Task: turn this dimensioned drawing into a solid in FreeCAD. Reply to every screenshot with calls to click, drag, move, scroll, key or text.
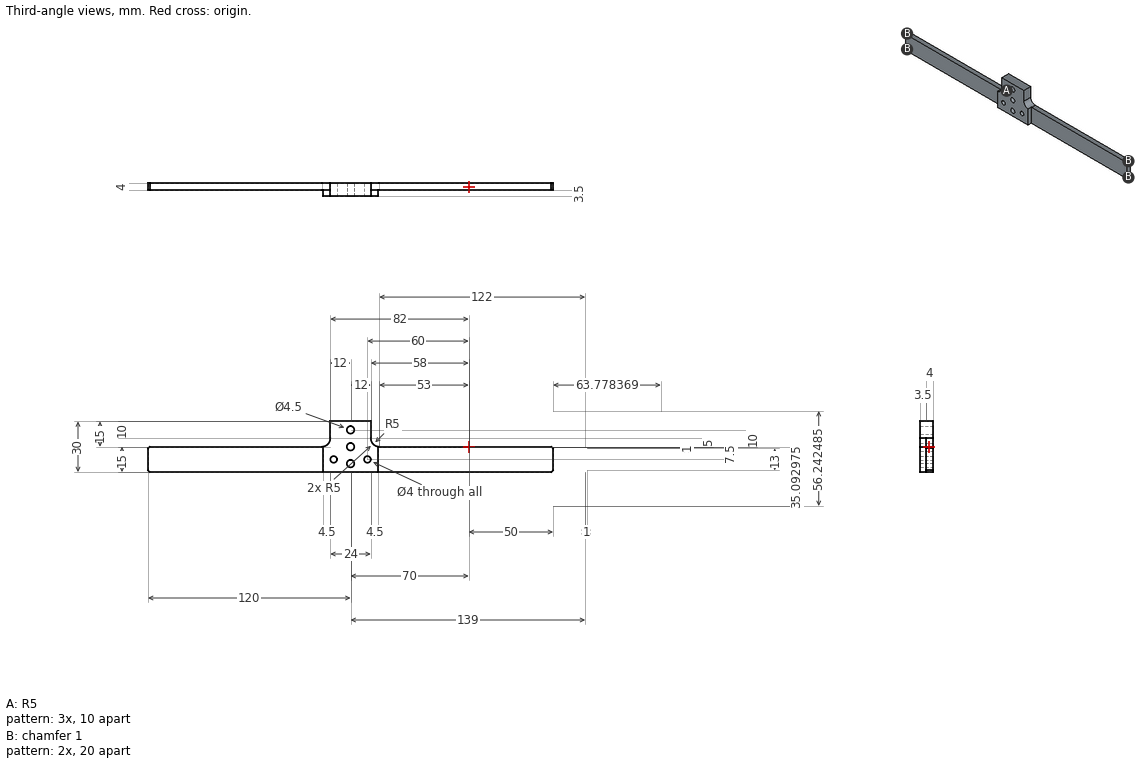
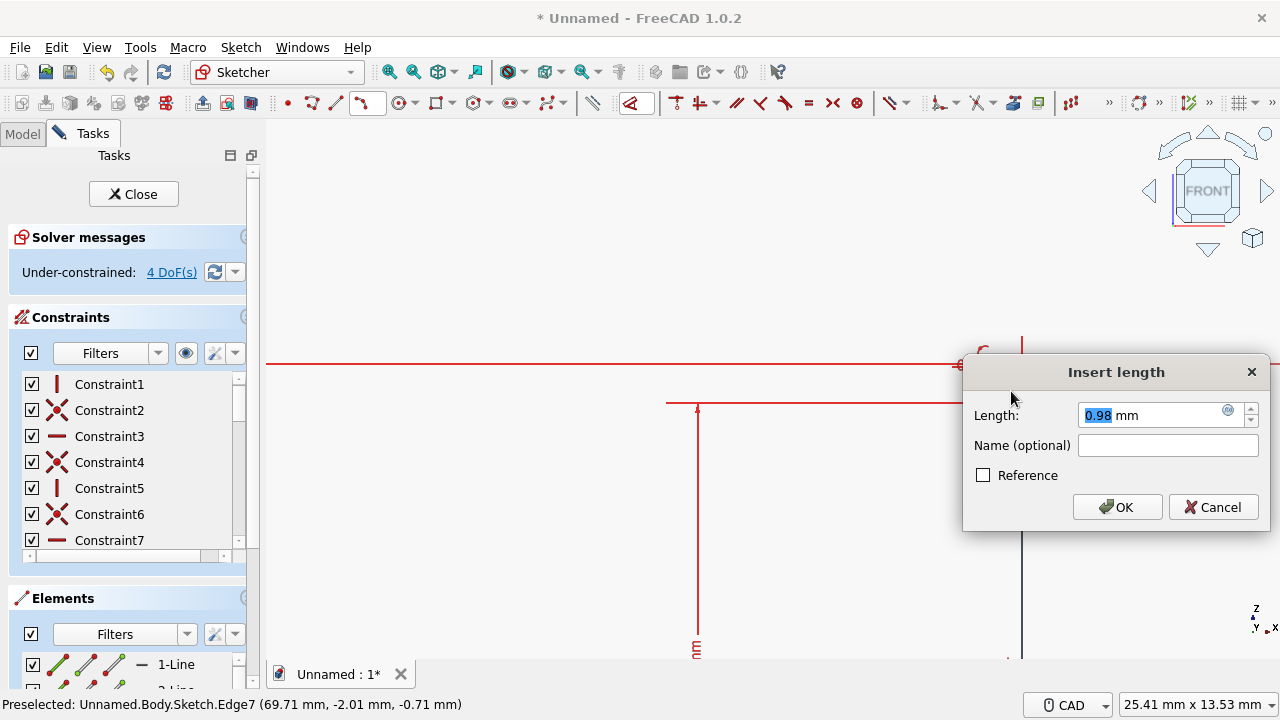
text(1)
key(Return)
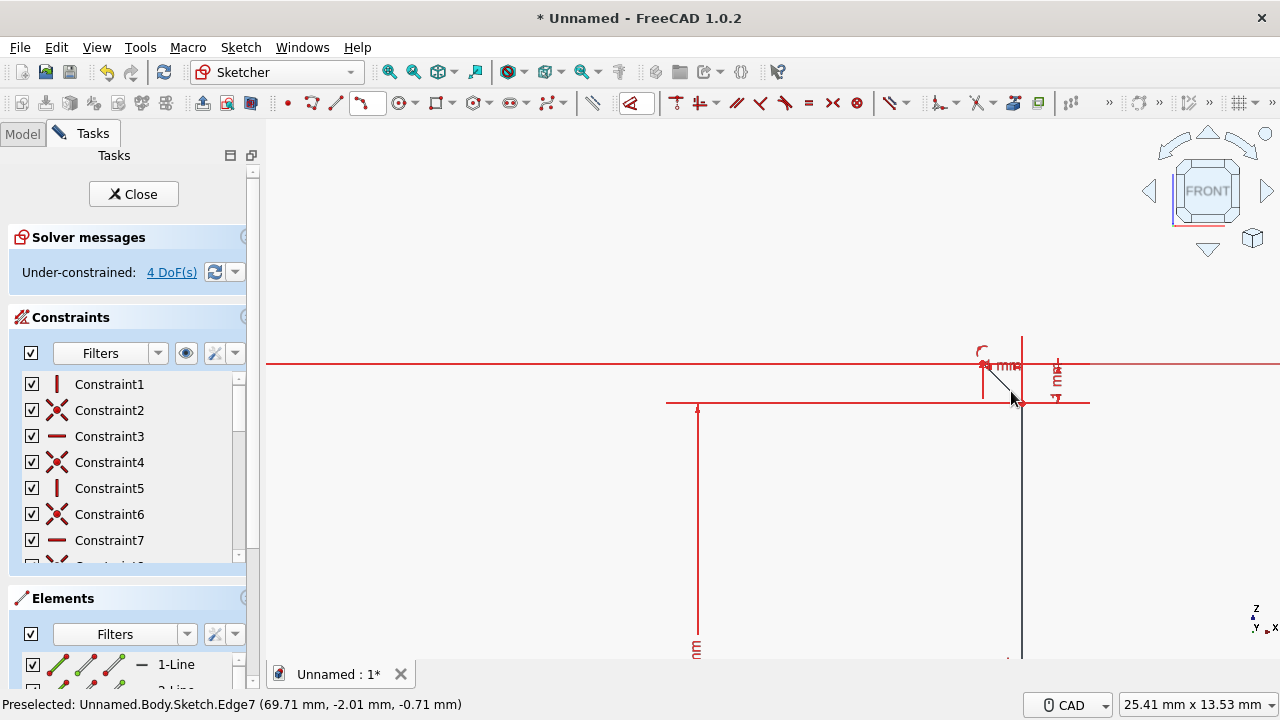
scroll(1013, 392, down, 11)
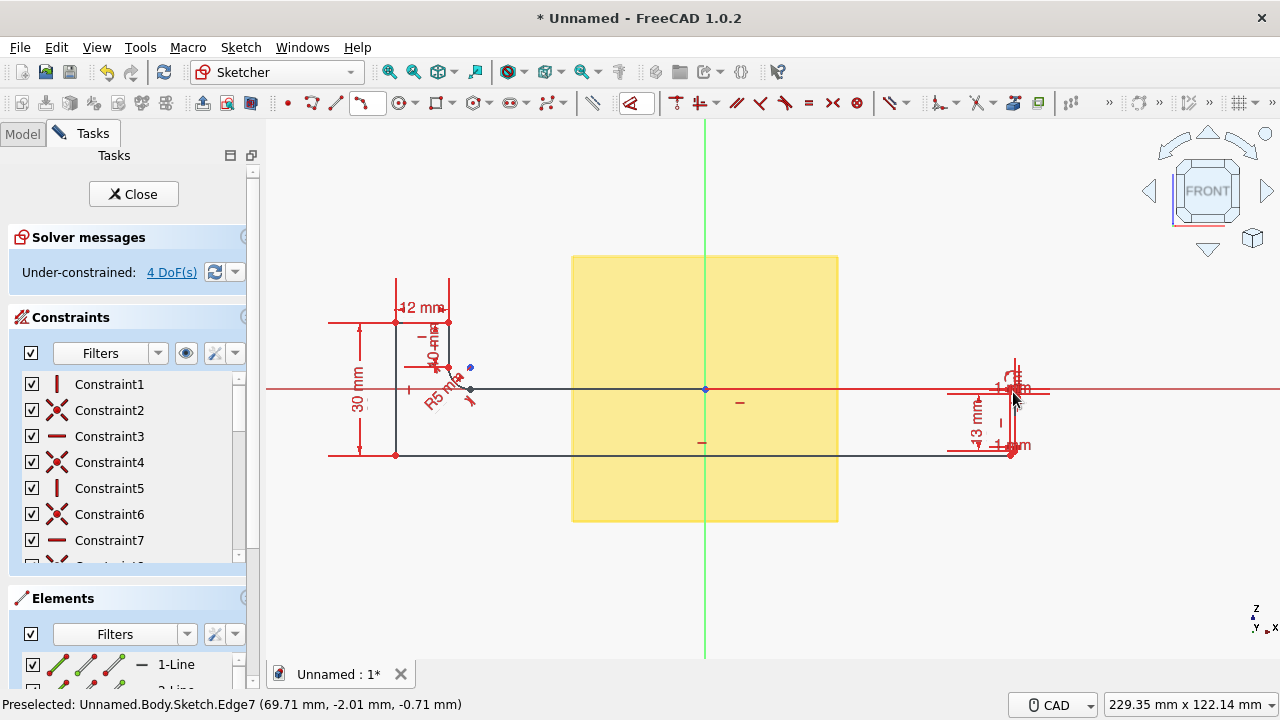
click(580, 456)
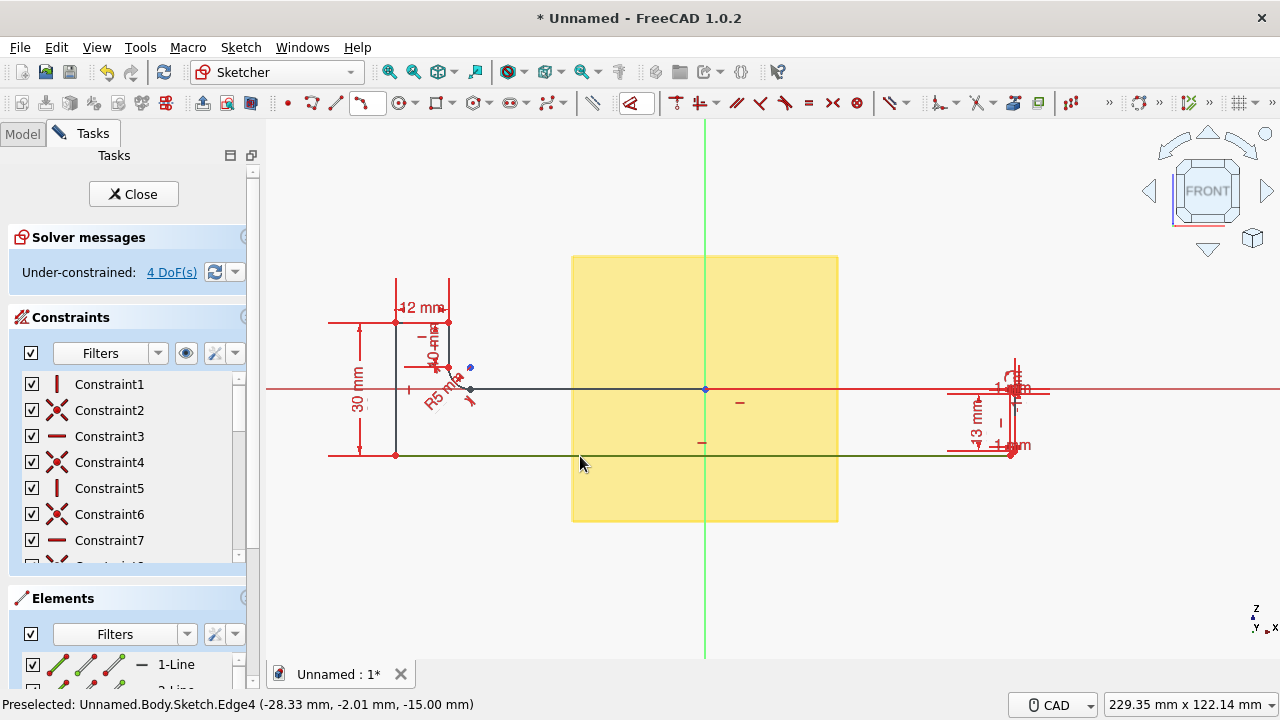
click(648, 104)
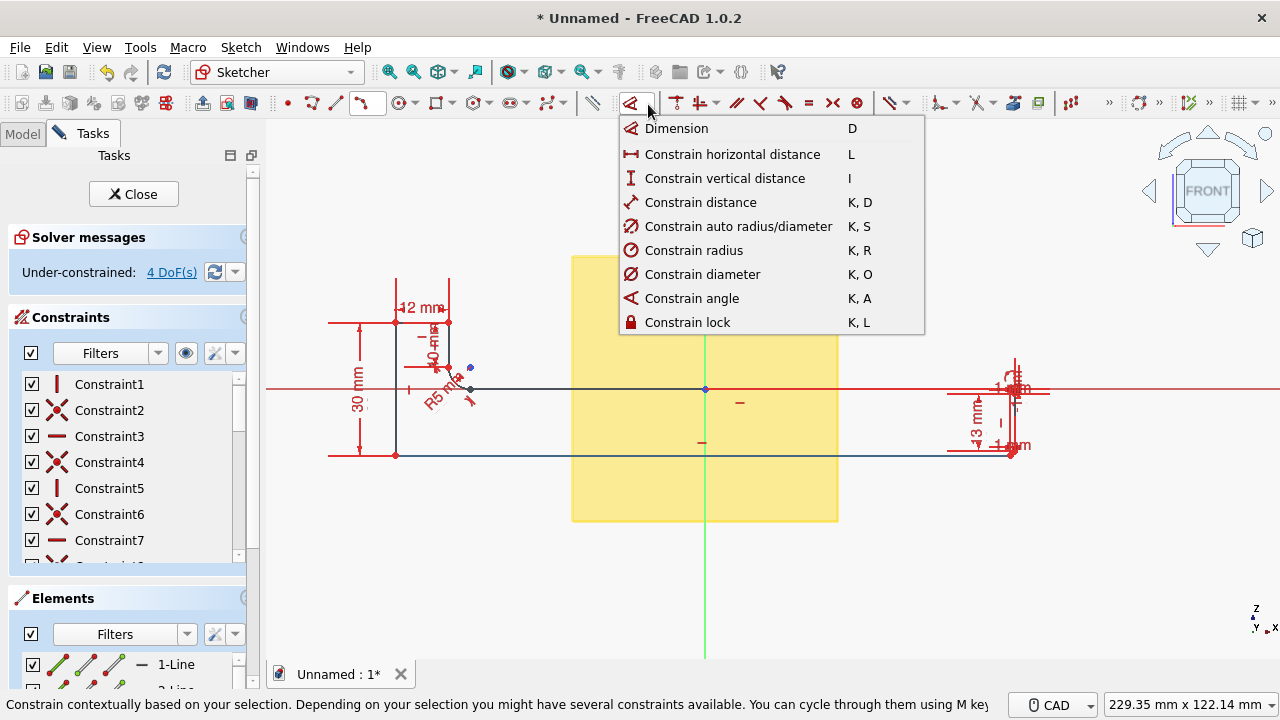
click(772, 154)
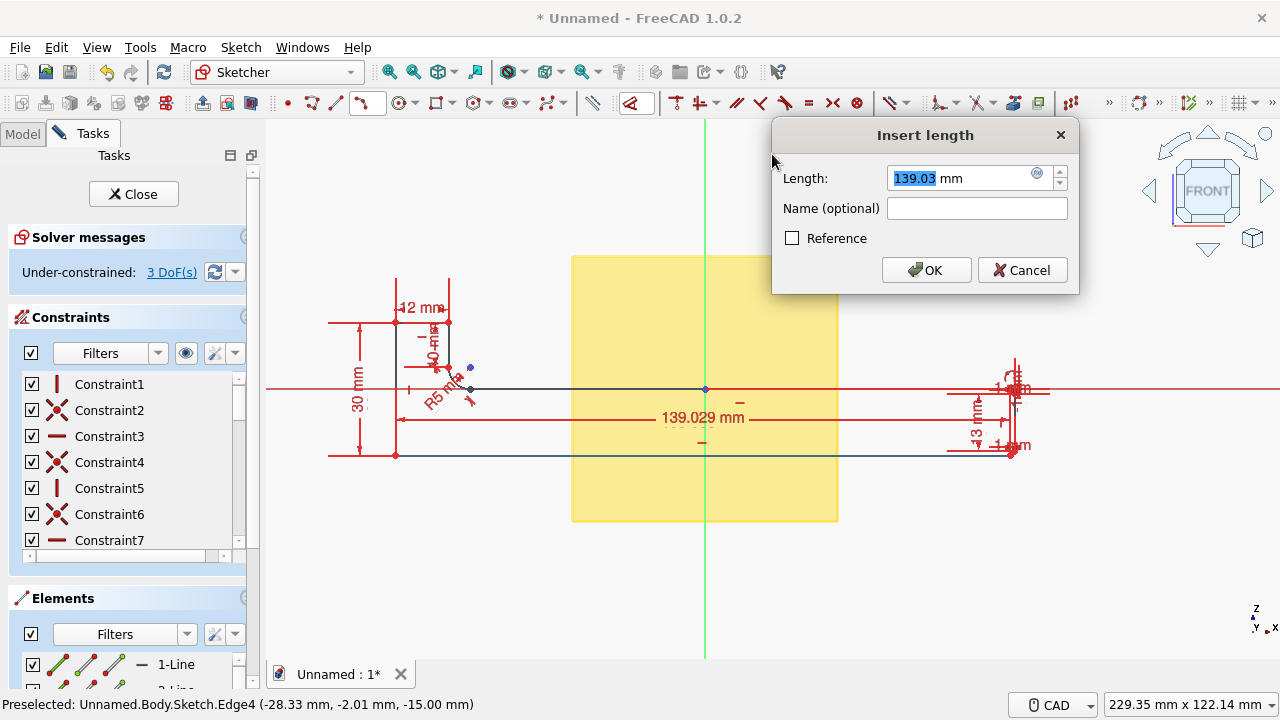
text(139)
key(Return)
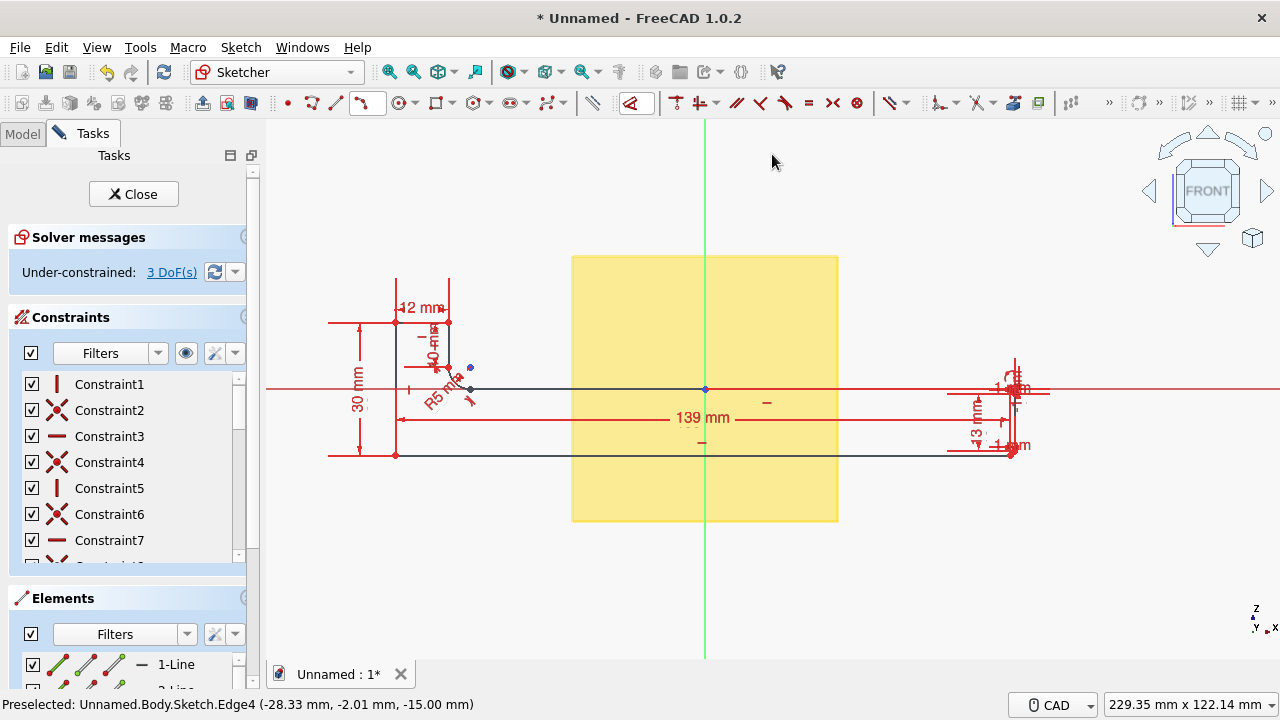
click(848, 389)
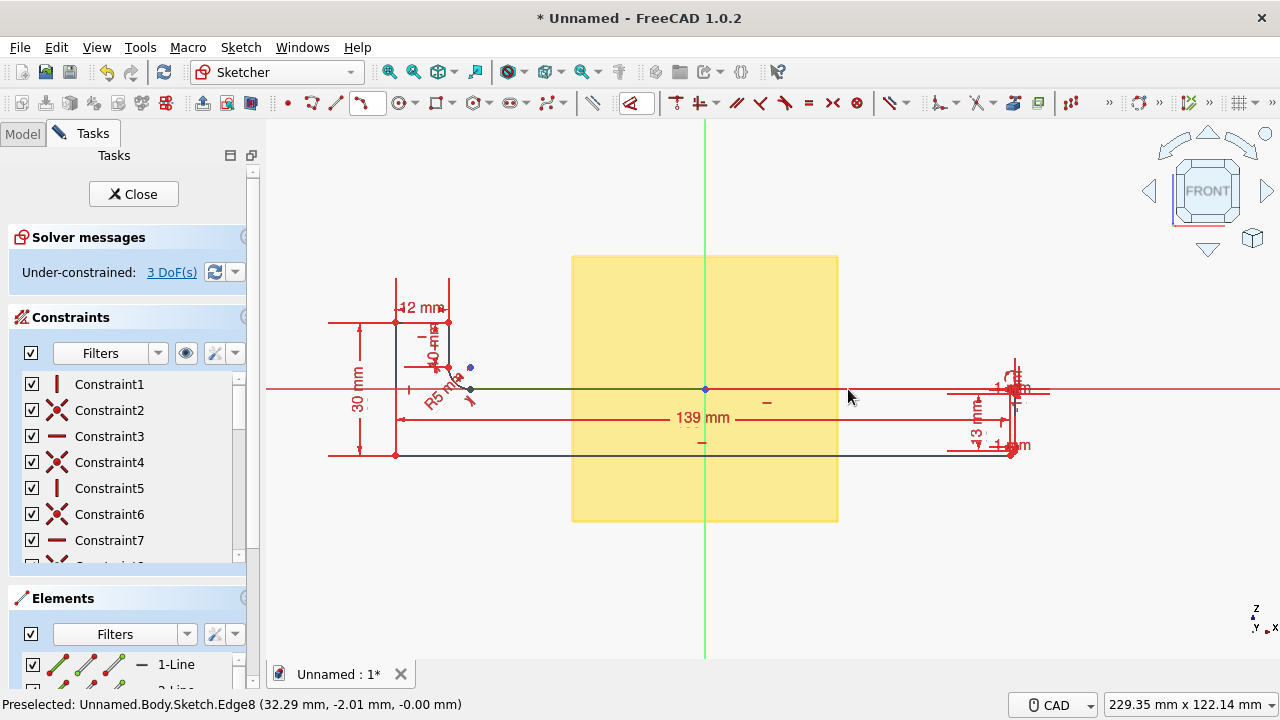
click(648, 104)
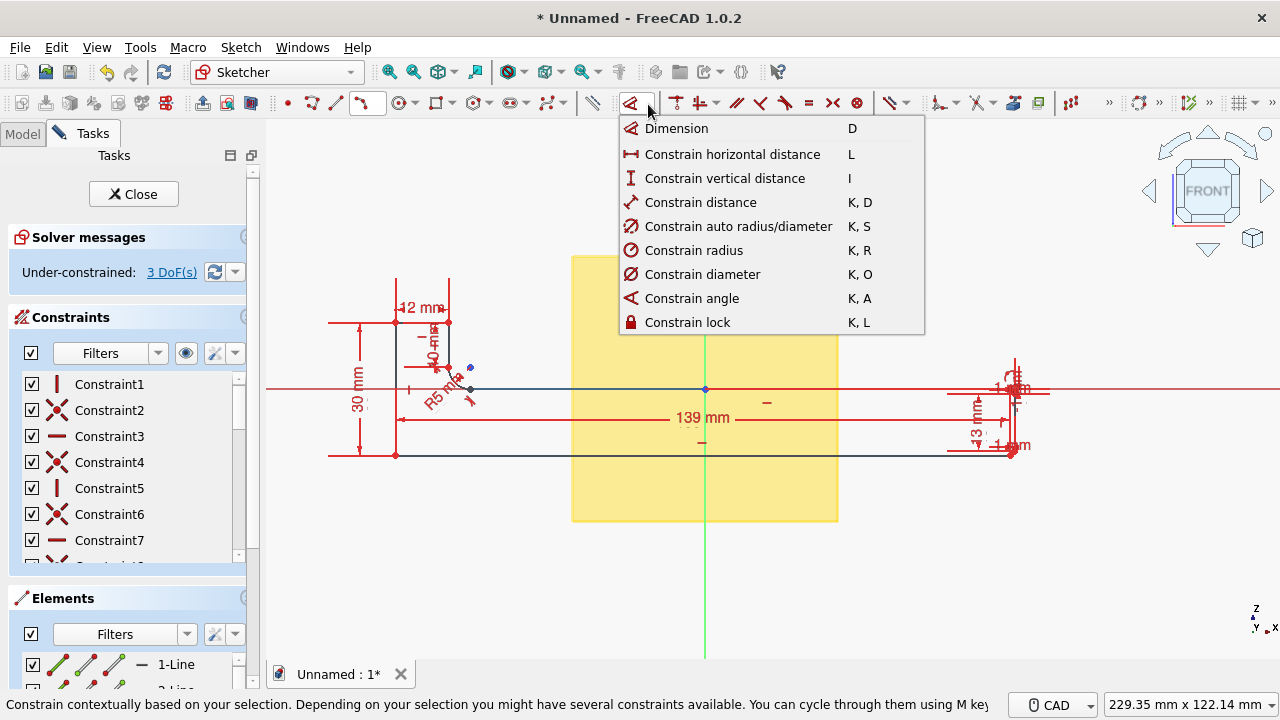
click(772, 154)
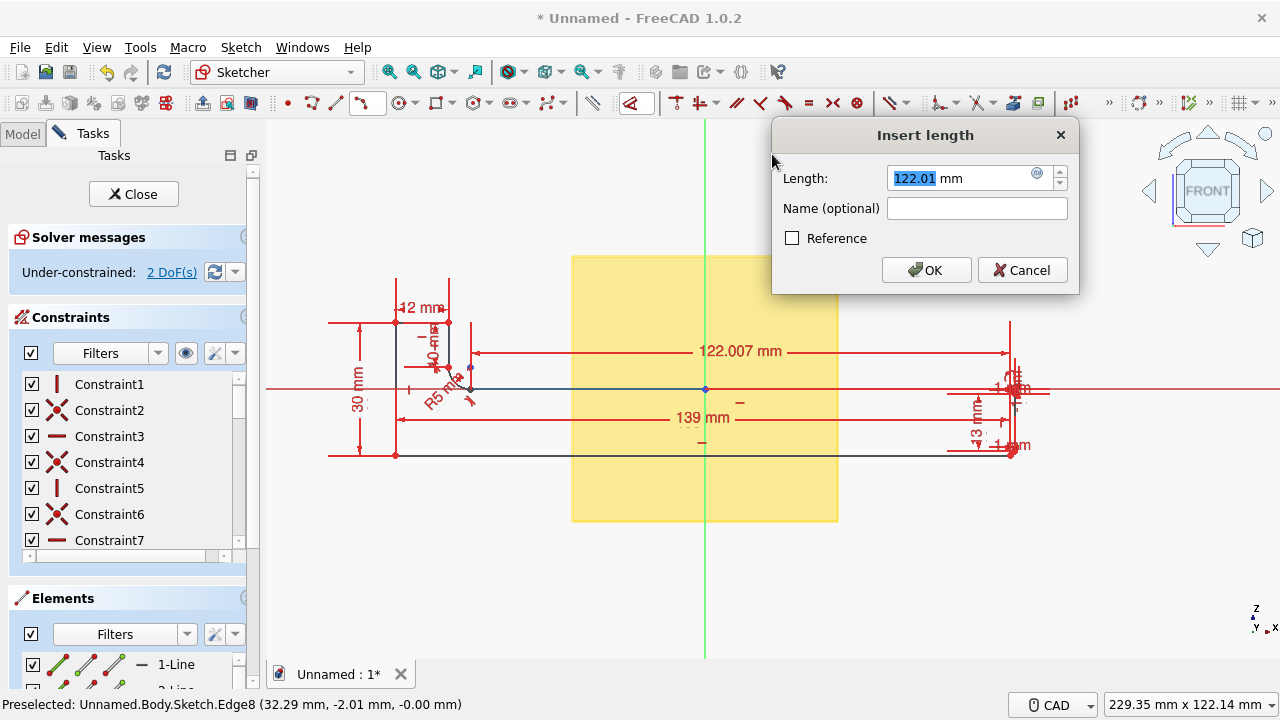
text(122)
key(Return)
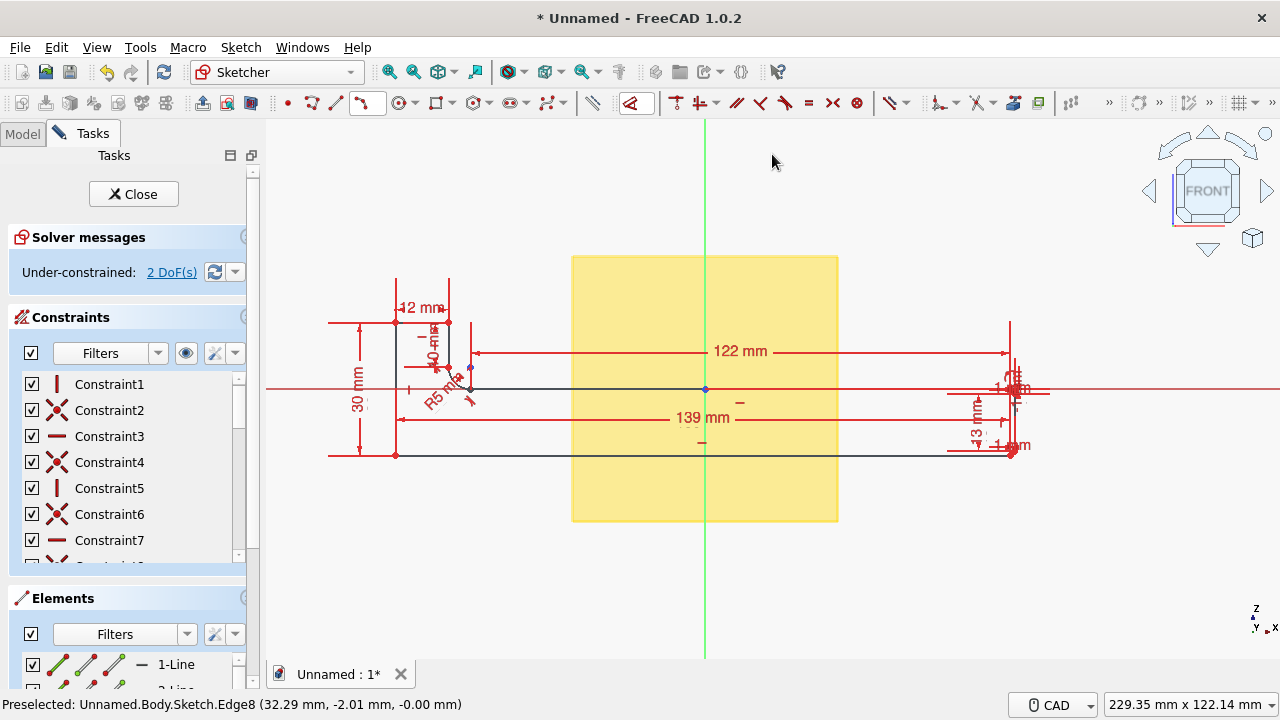
click(449, 367)